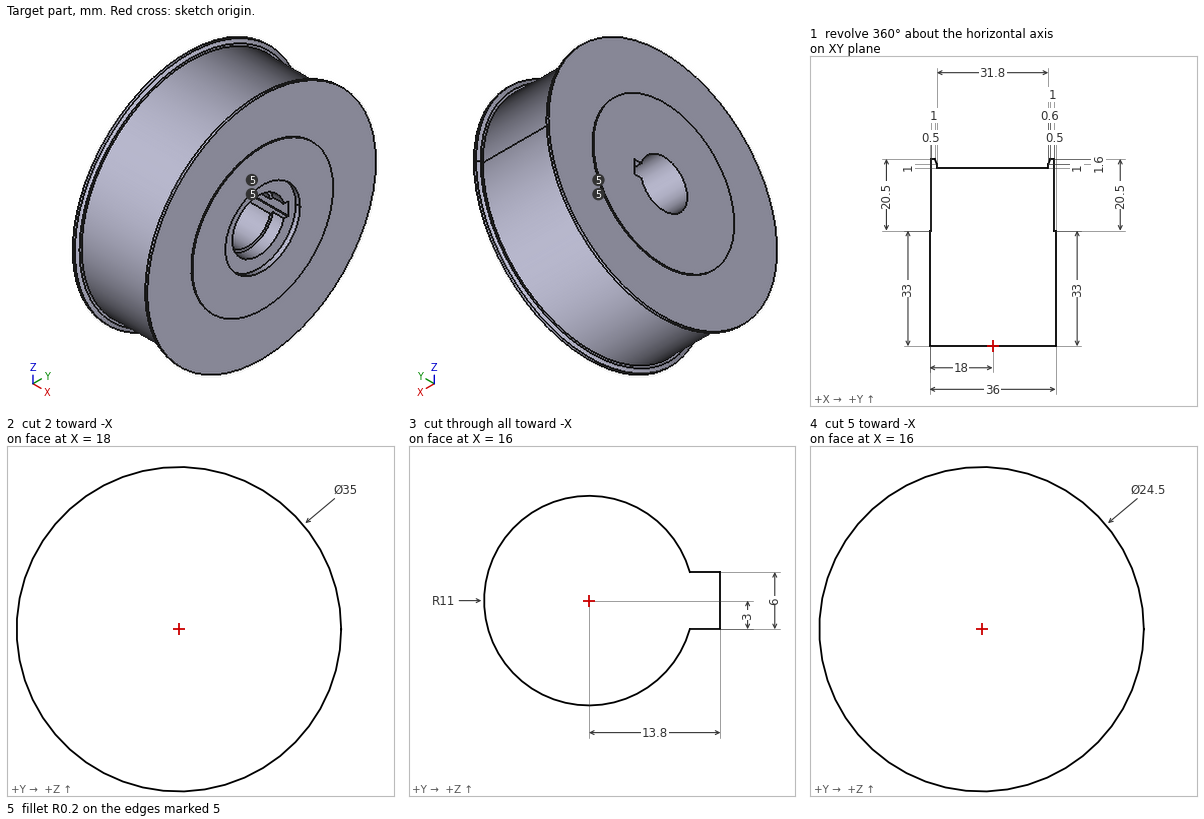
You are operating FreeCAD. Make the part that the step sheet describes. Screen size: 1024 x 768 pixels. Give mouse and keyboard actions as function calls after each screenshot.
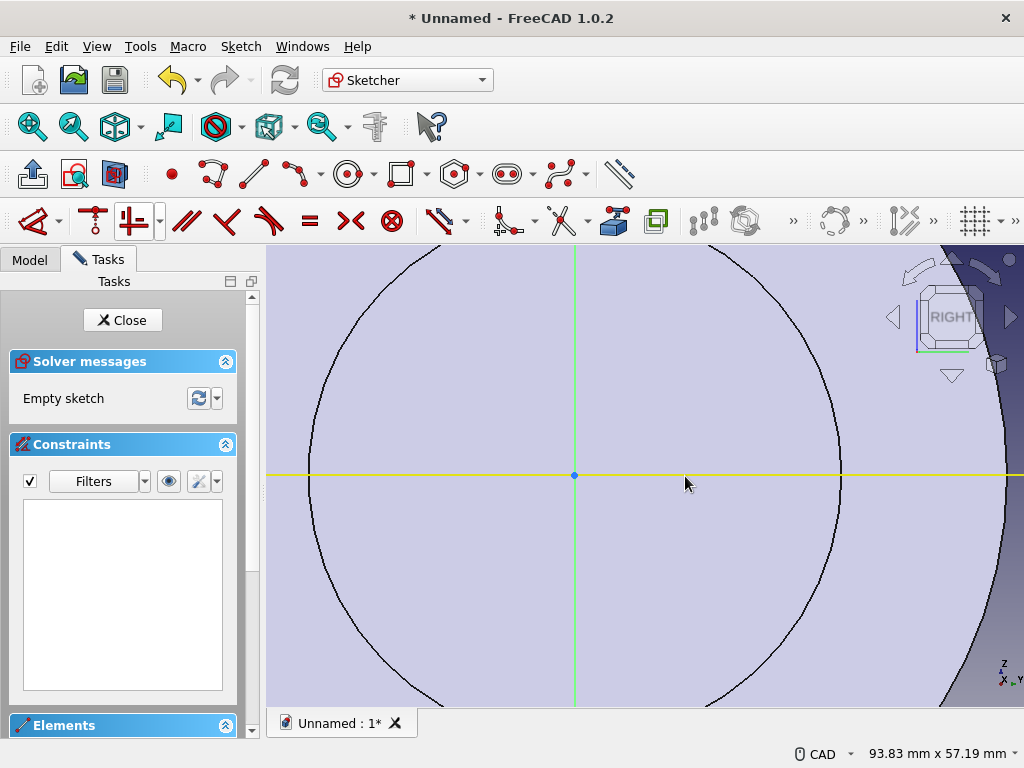
key(g)
key(c)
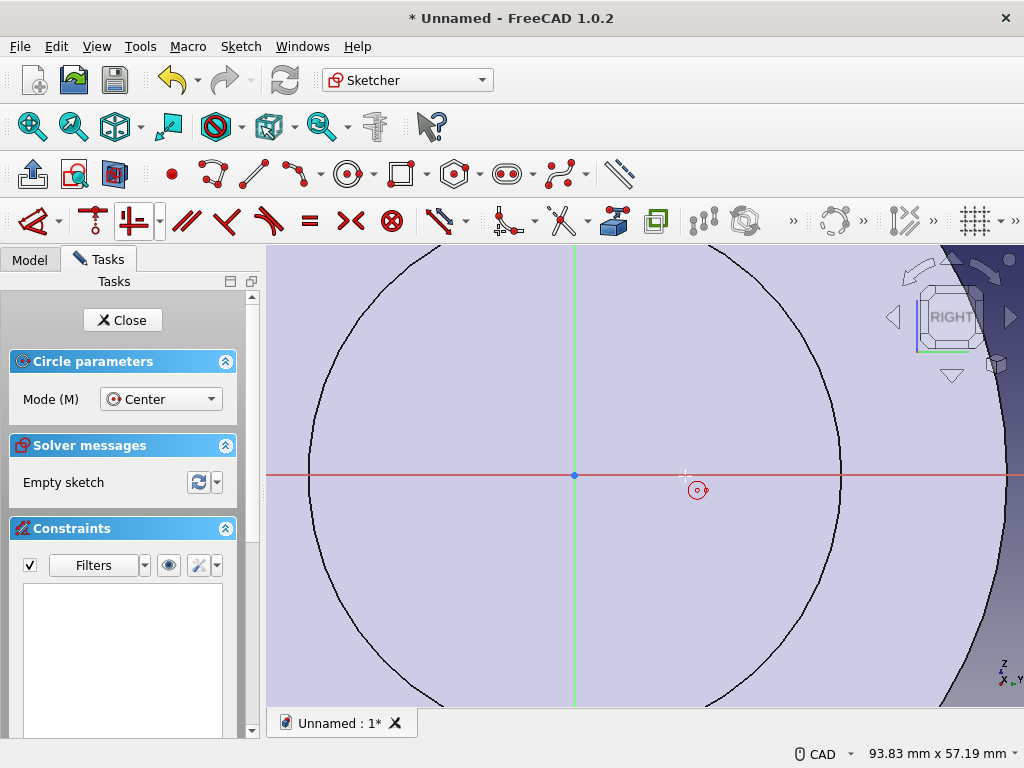
click(575, 475)
click(675, 375)
key(Escape)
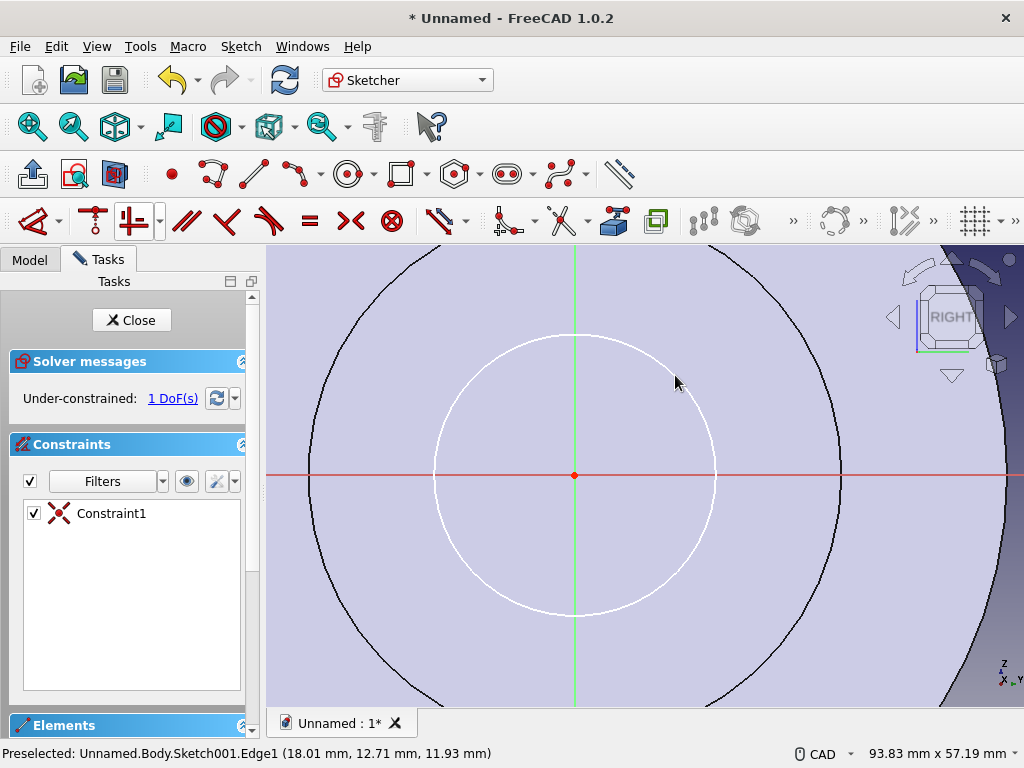
click(32, 222)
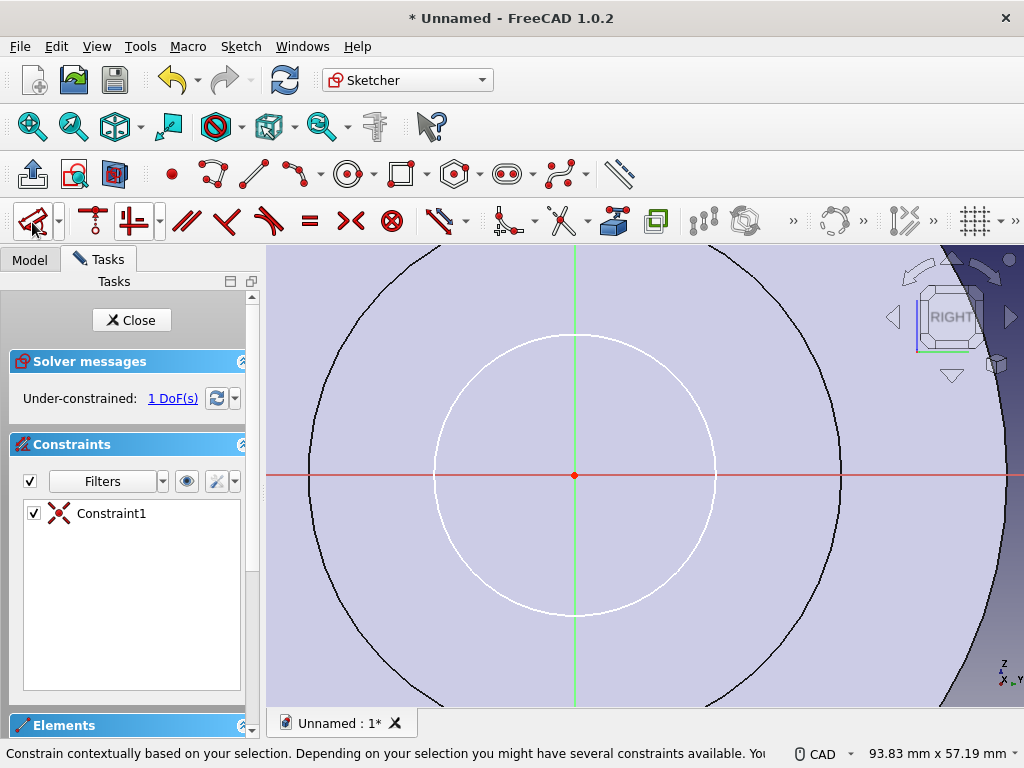
click(674, 375)
click(696, 352)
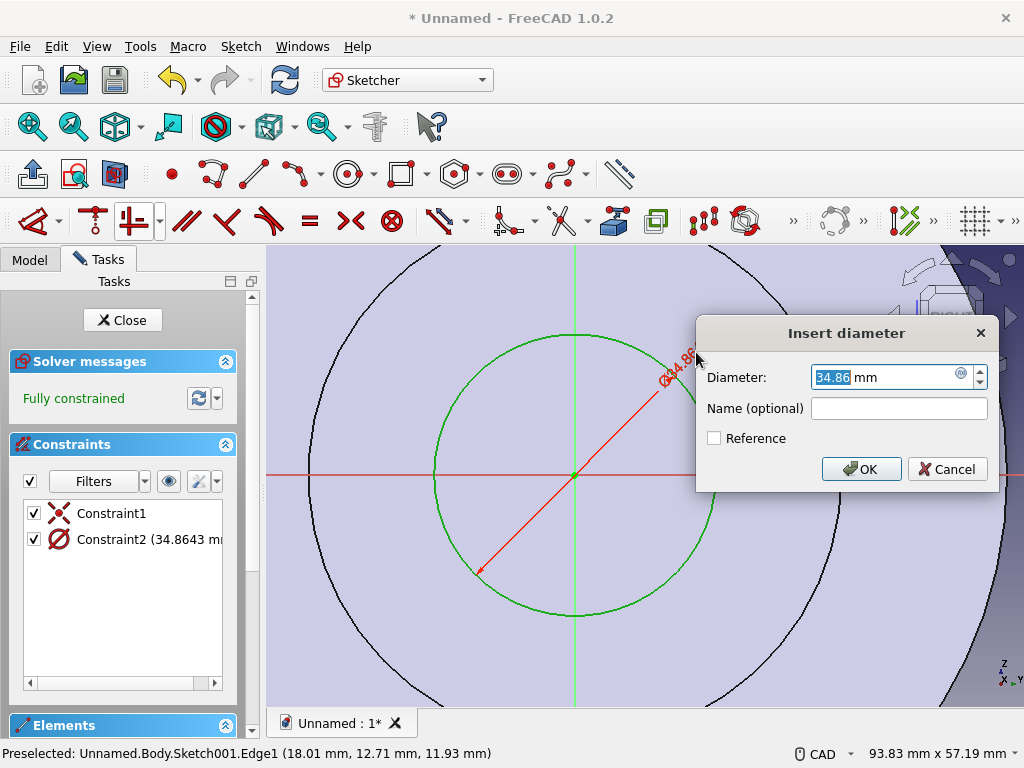
text(35)
key(Return)
key(Escape)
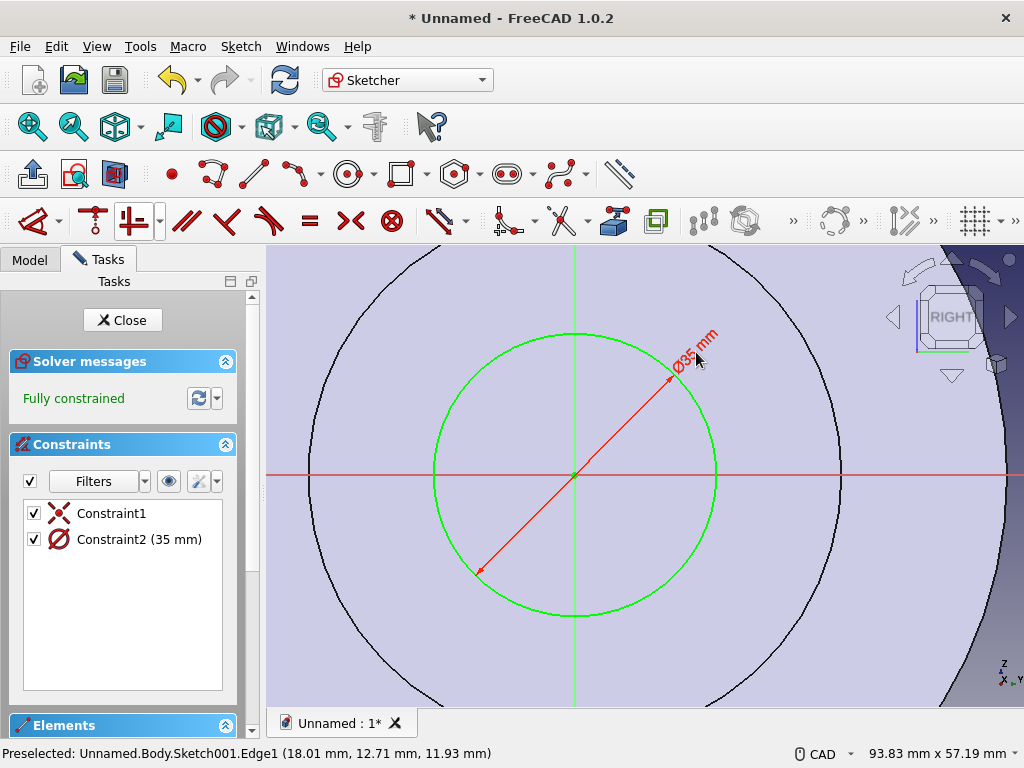
click(123, 320)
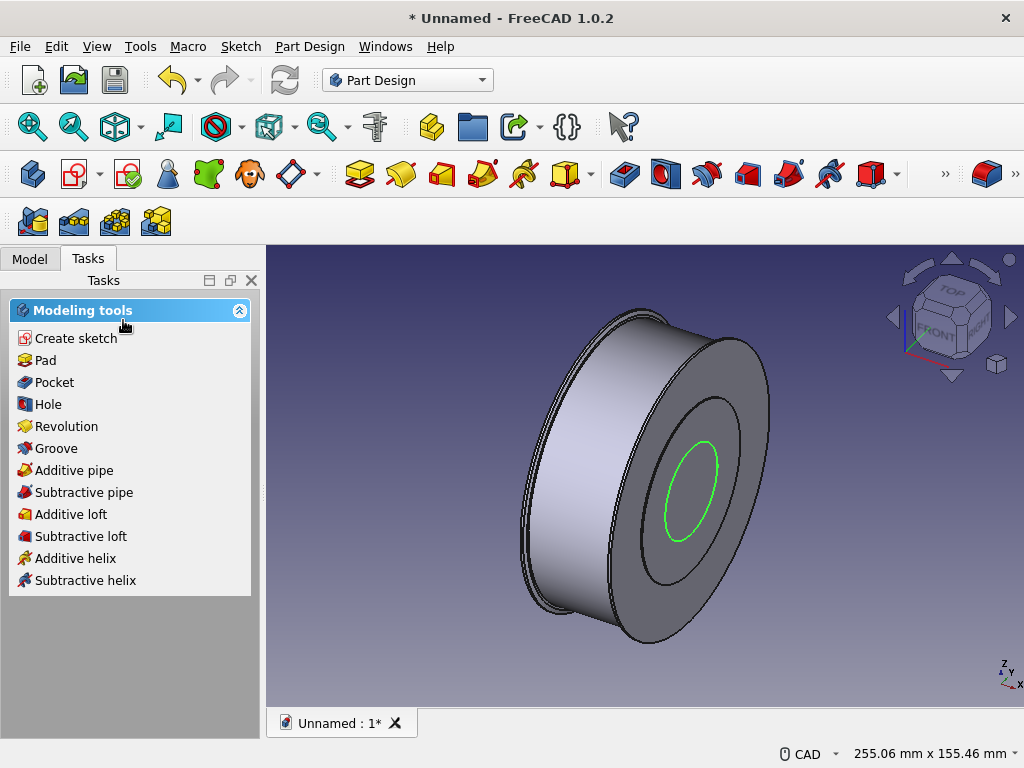
click(625, 174)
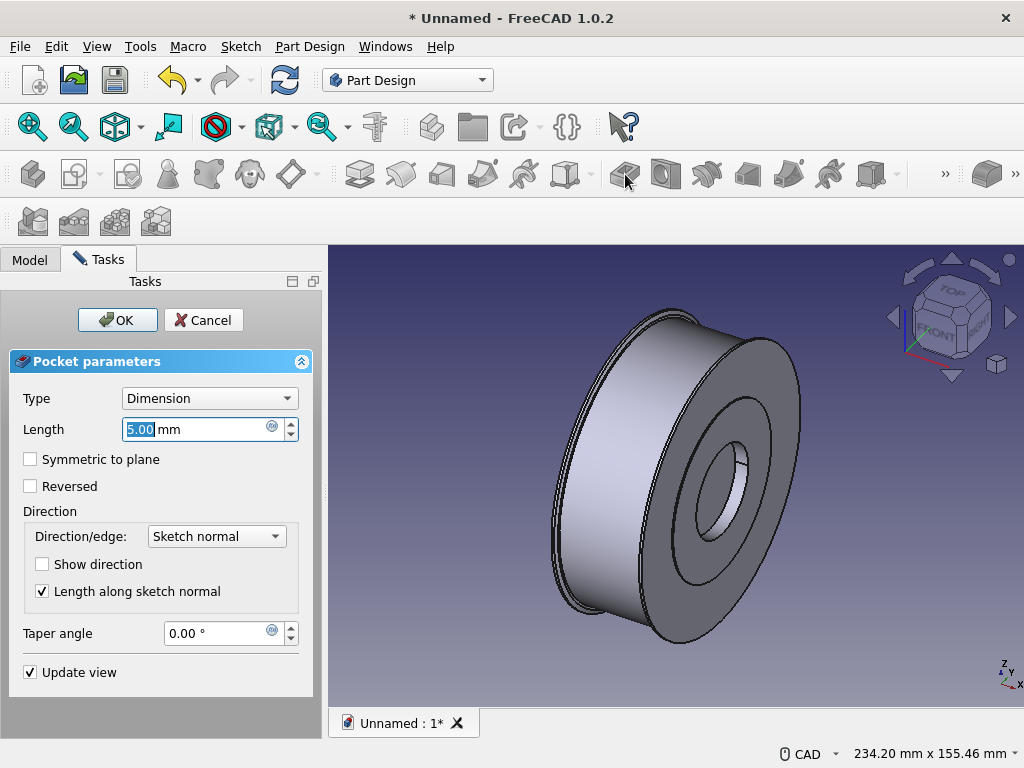
text(2)
key(Tab)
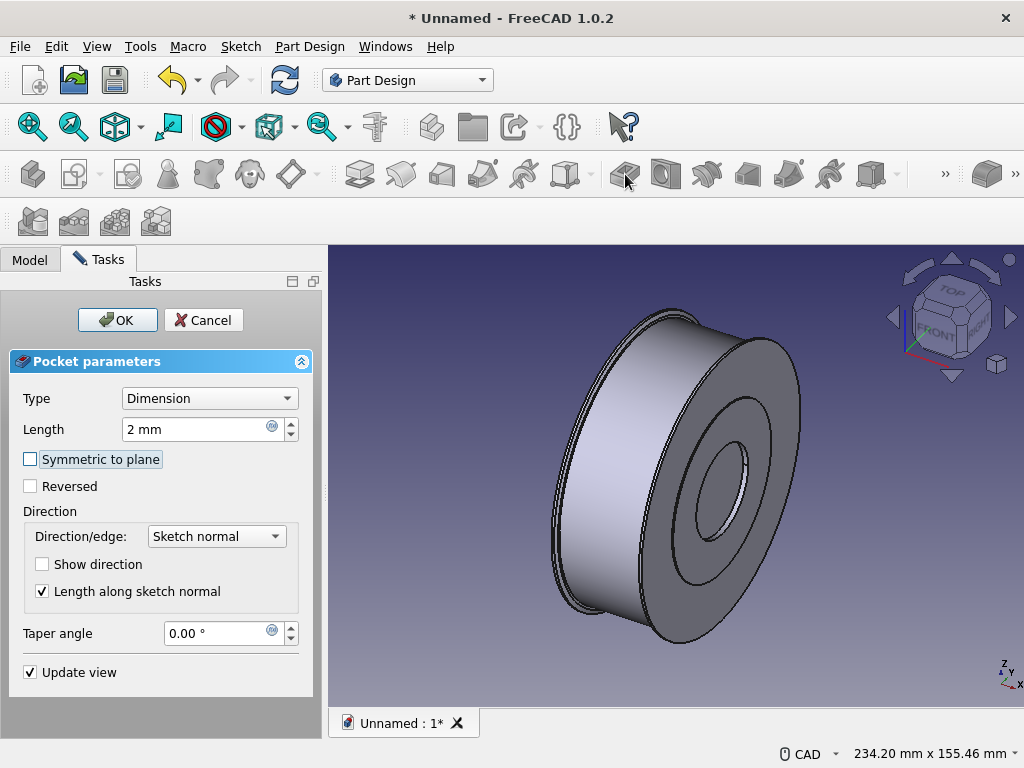
click(118, 320)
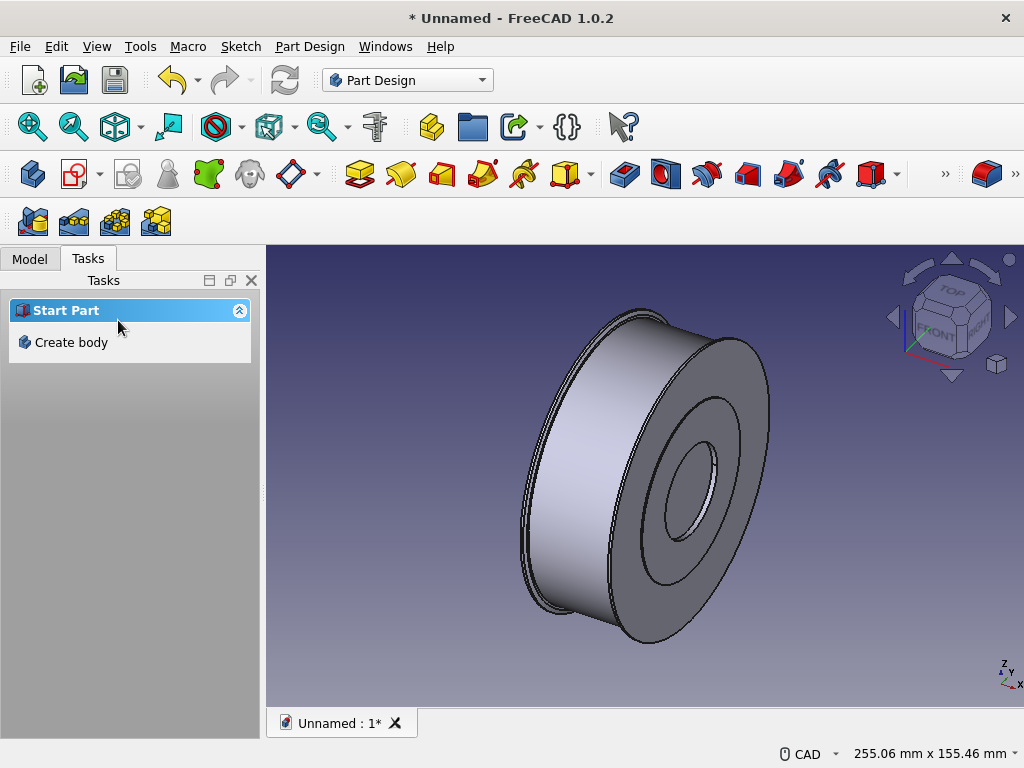
click(686, 489)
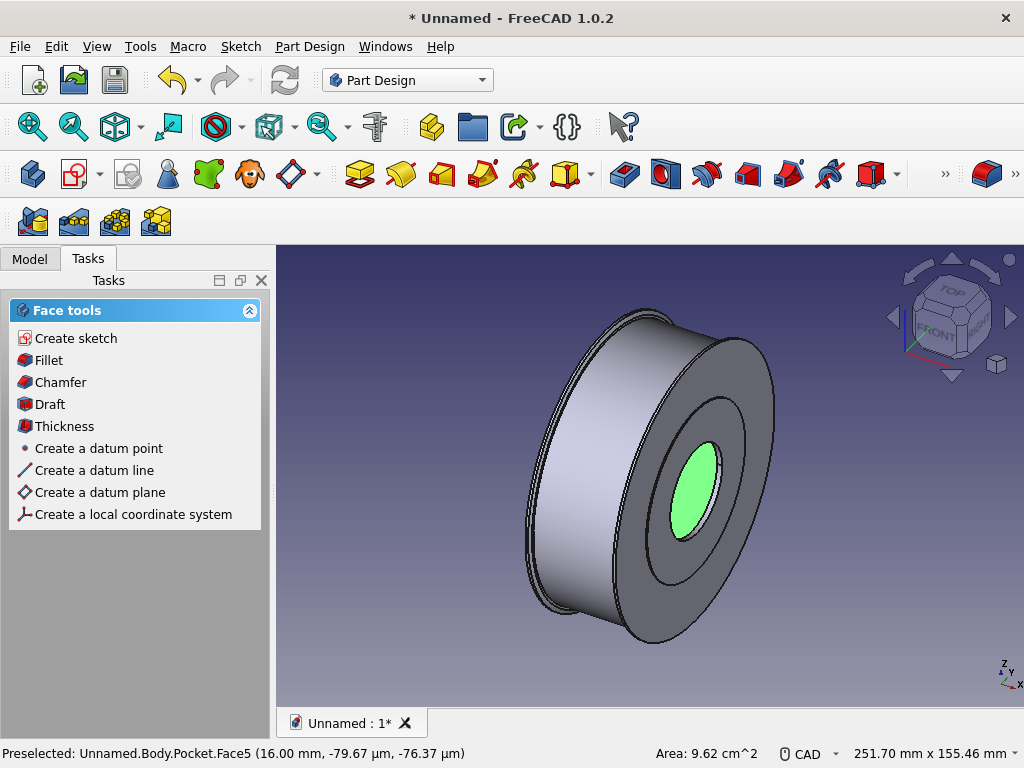
click(74, 174)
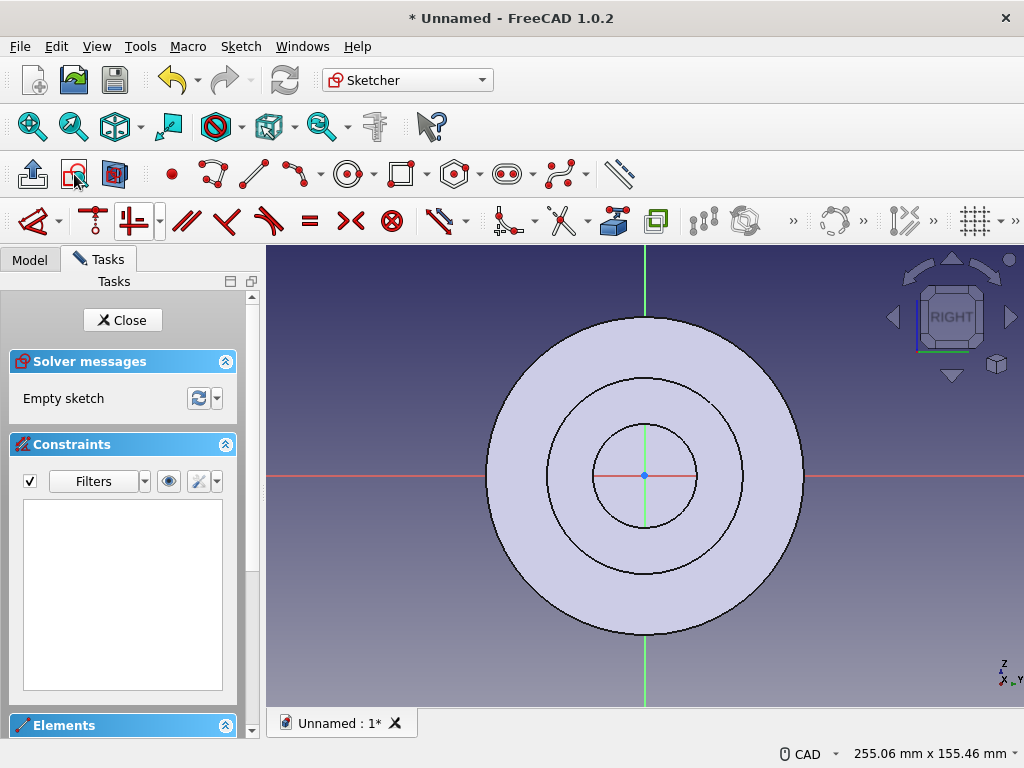
key(q)
key(s)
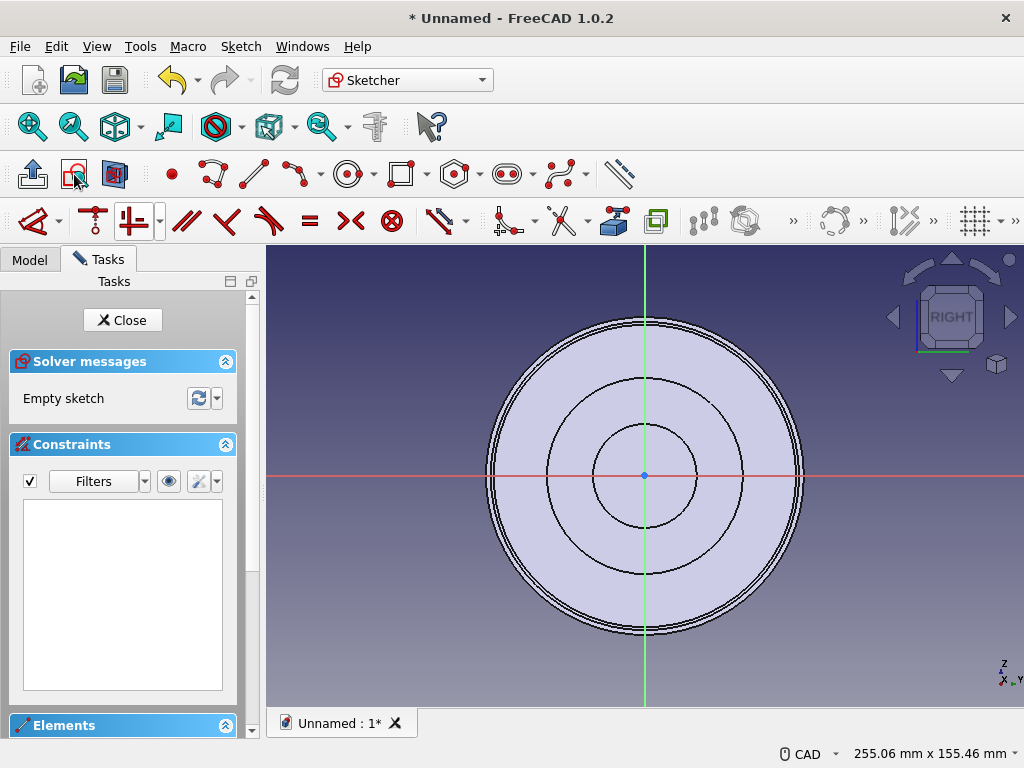
scroll(667, 476, up, 8)